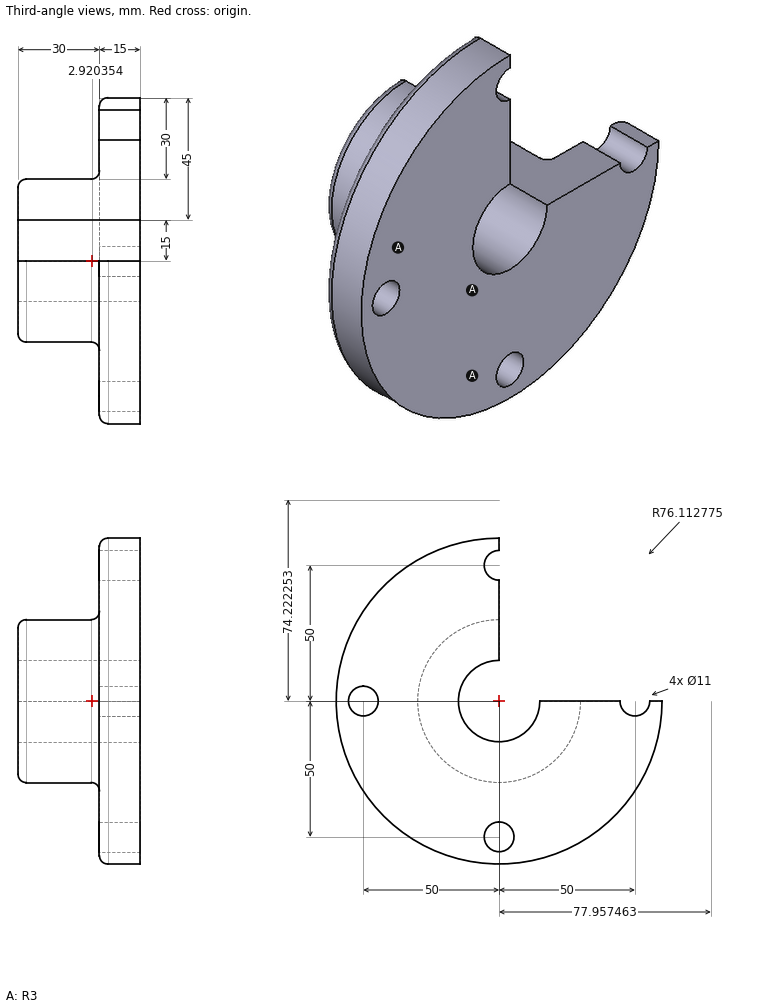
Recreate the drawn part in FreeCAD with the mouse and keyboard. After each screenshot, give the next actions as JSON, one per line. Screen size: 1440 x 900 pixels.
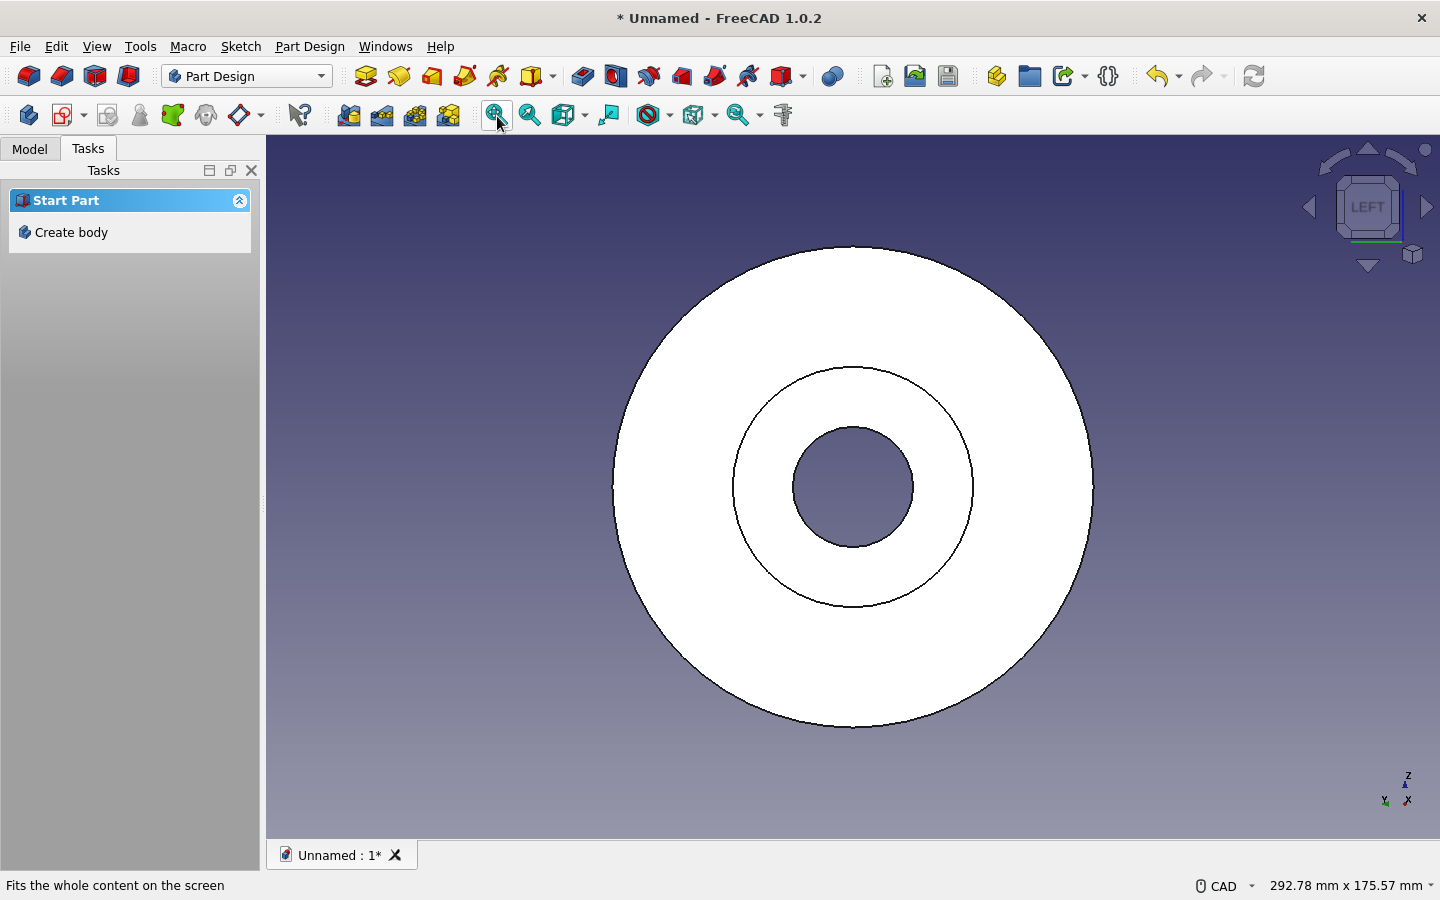
{"action": "left_click", "coordinate": [990, 623]}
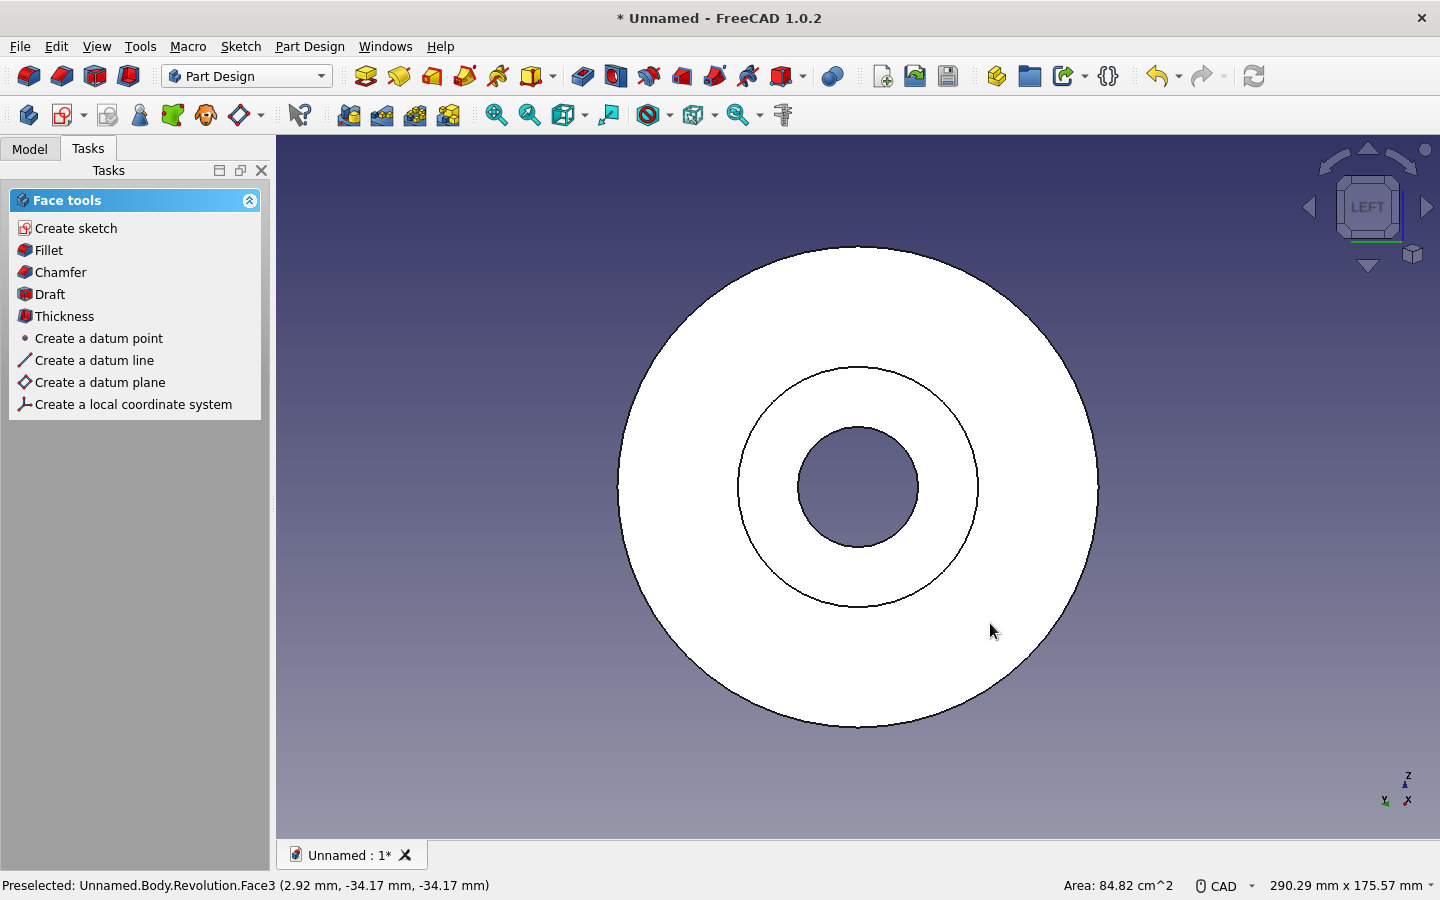
{"action": "left_click", "coordinate": [62, 116]}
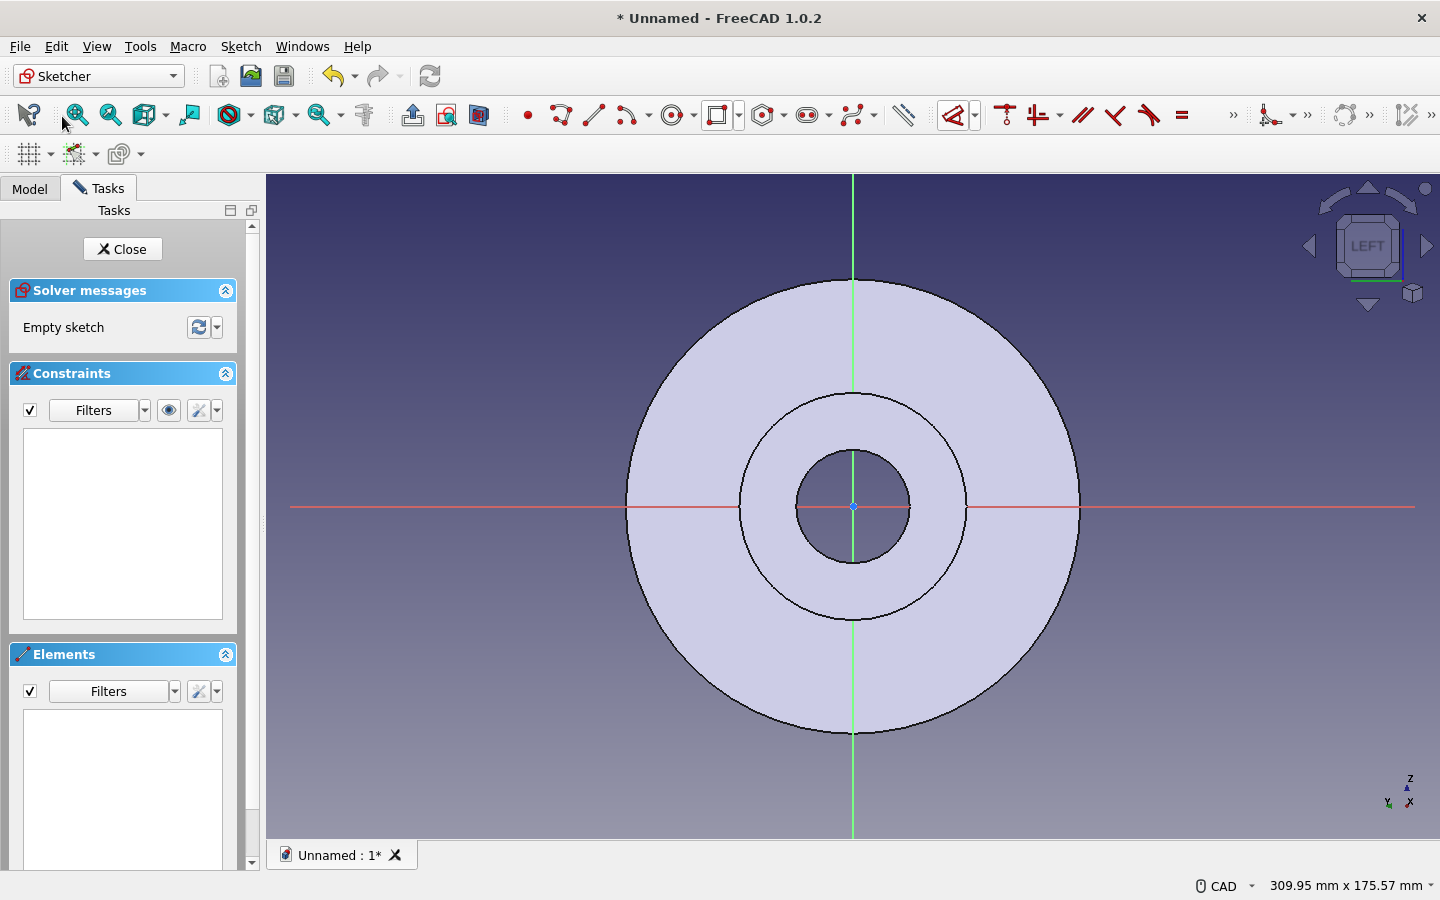
{"action": "left_click", "coordinate": [479, 116]}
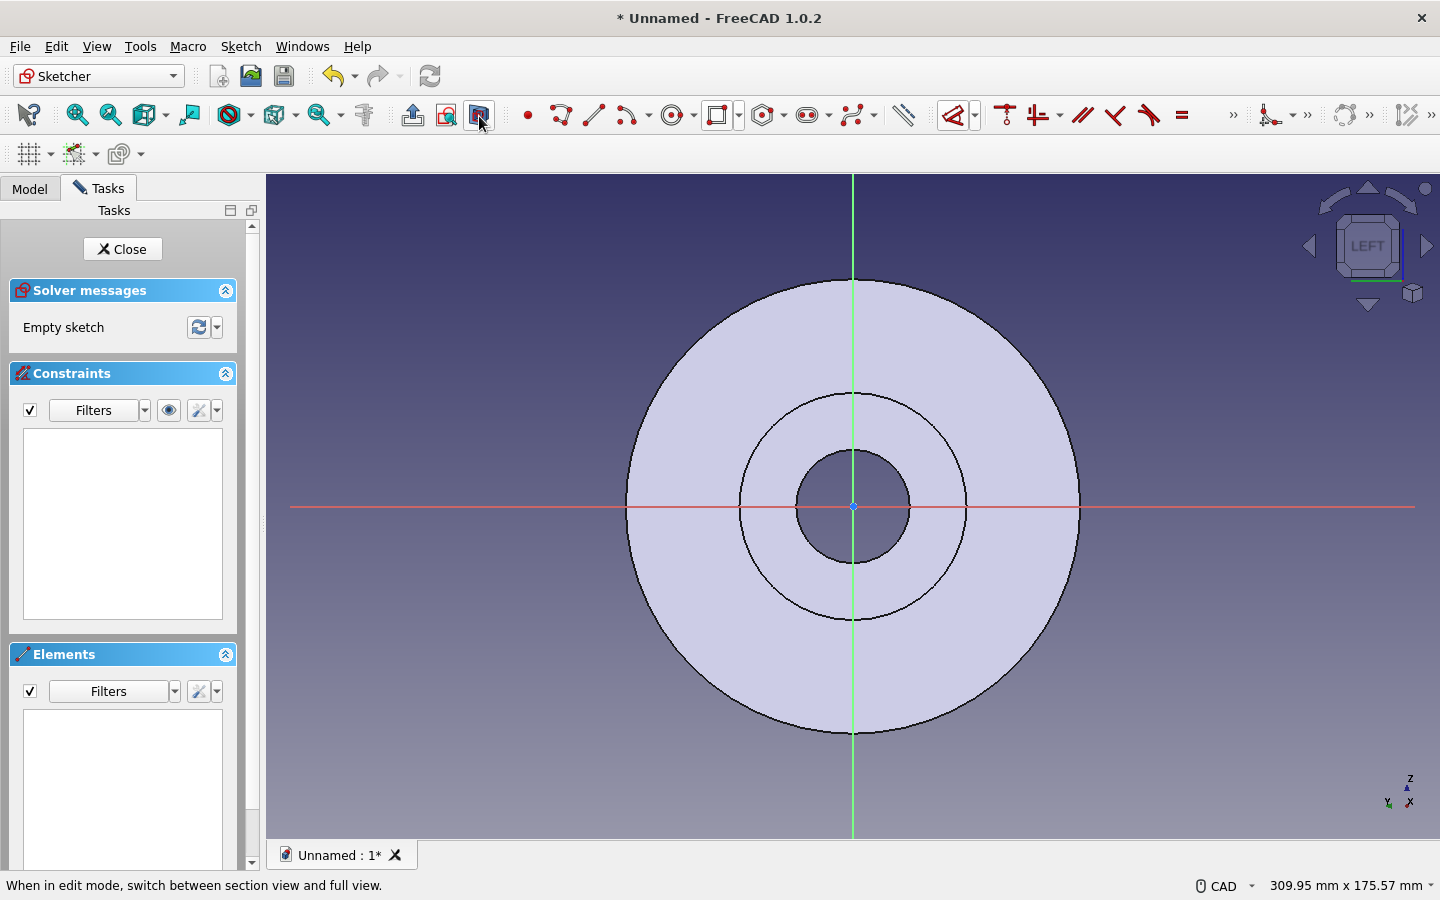
{"action": "left_click", "coordinate": [672, 116]}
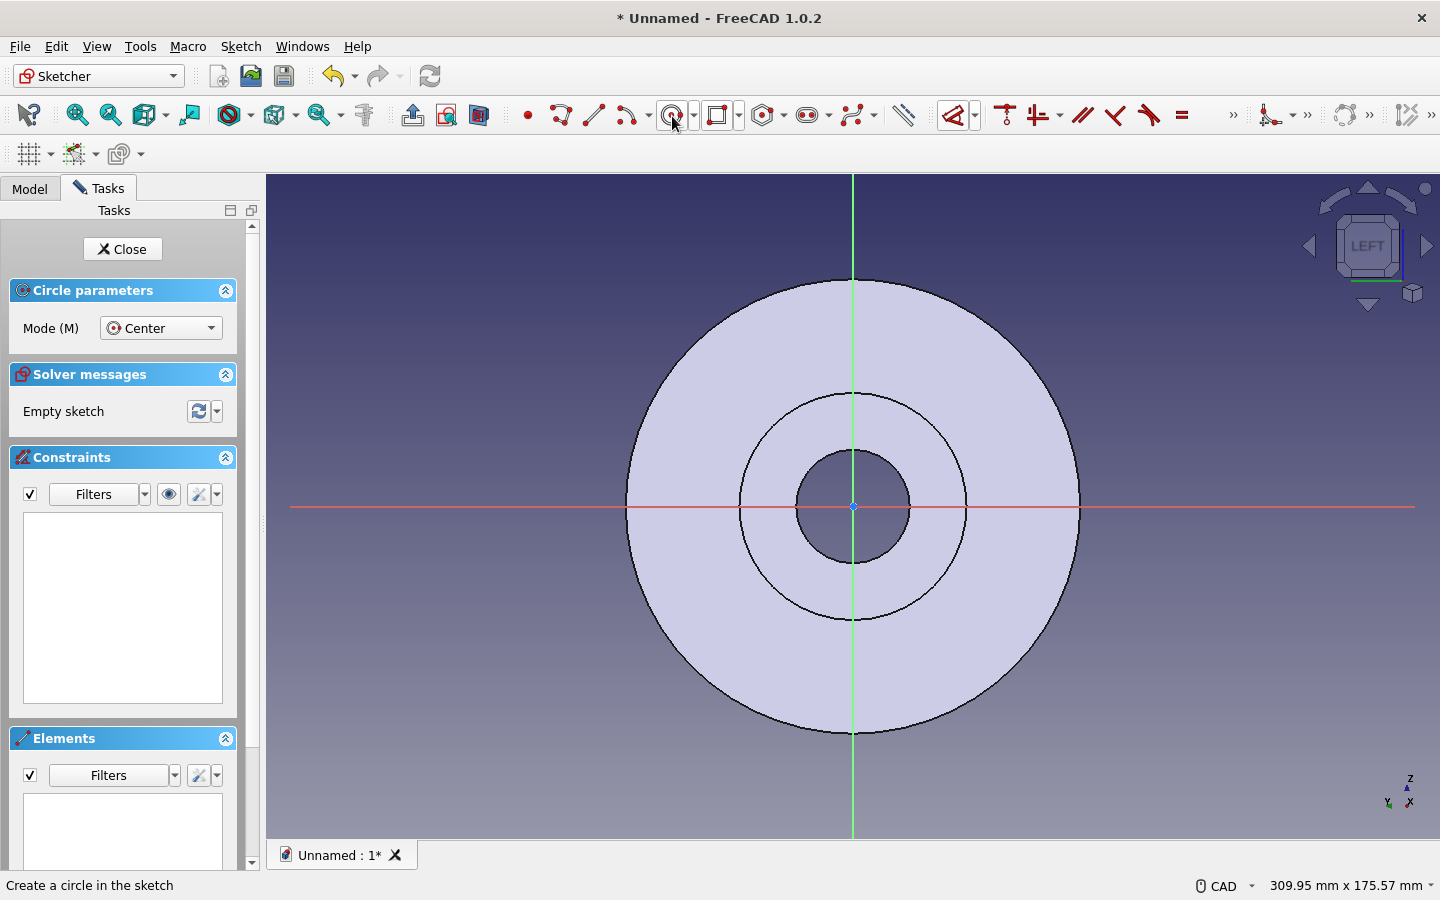
{"action": "left_click", "coordinate": [664, 506]}
{"action": "left_click", "coordinate": [678, 492]}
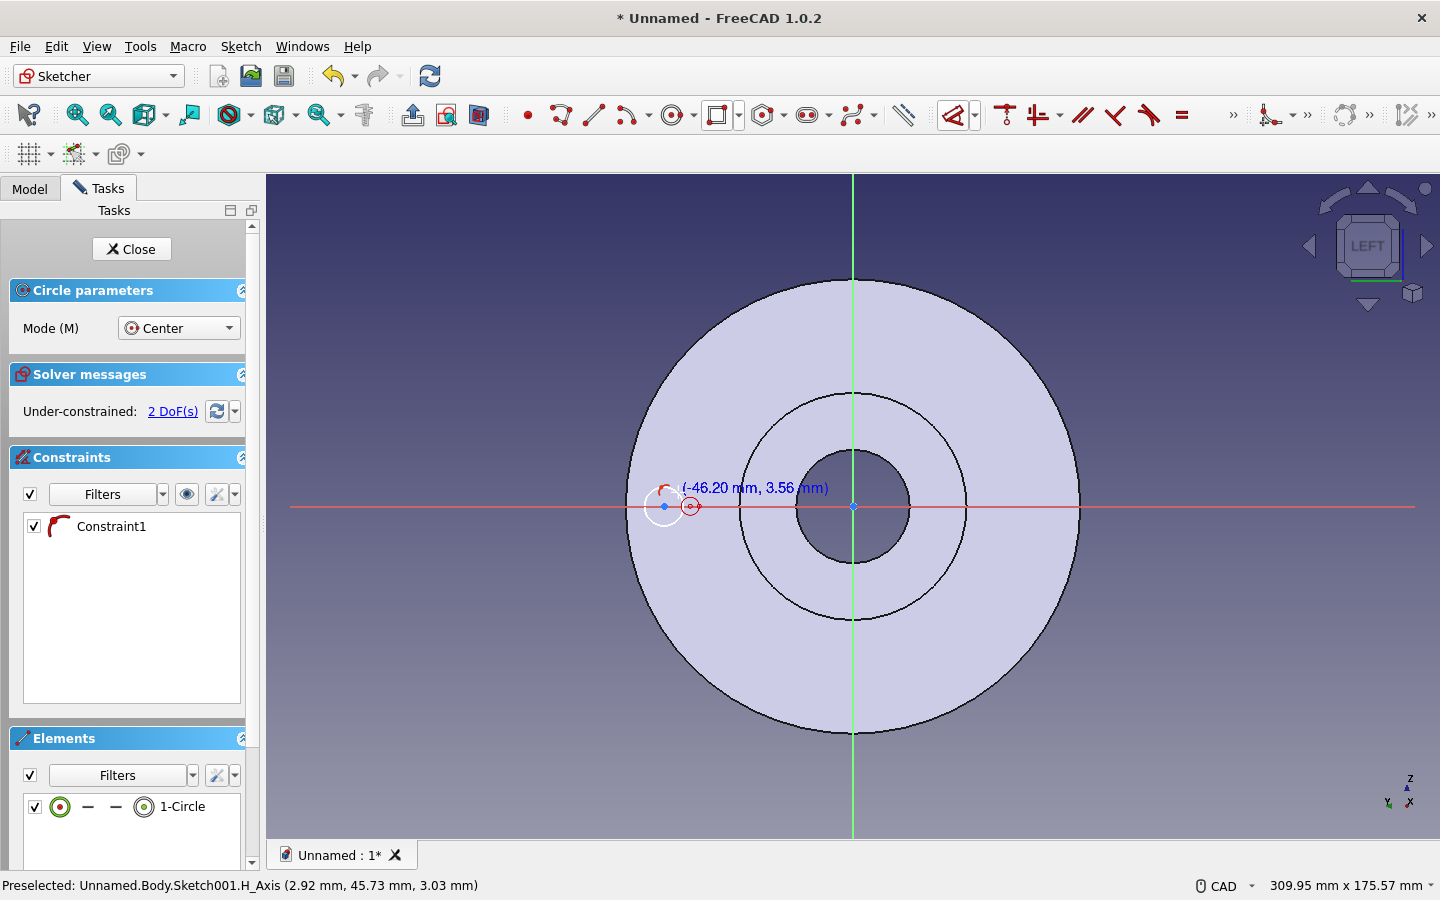
{"action": "left_click", "coordinate": [853, 317]}
{"action": "left_click", "coordinate": [868, 302]}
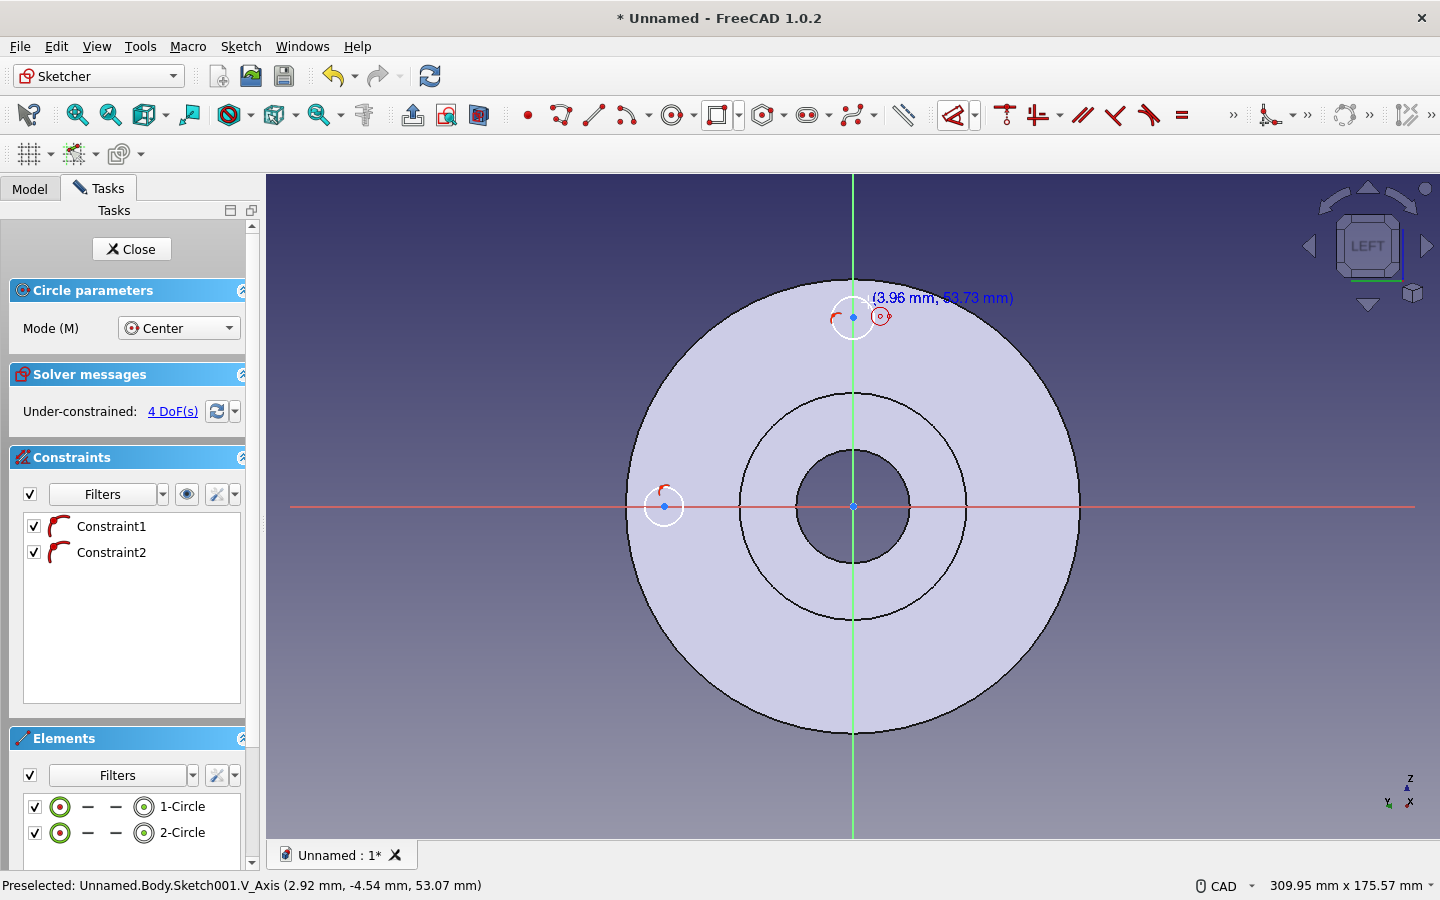
{"action": "left_click", "coordinate": [1042, 506]}
{"action": "left_click", "coordinate": [1057, 492]}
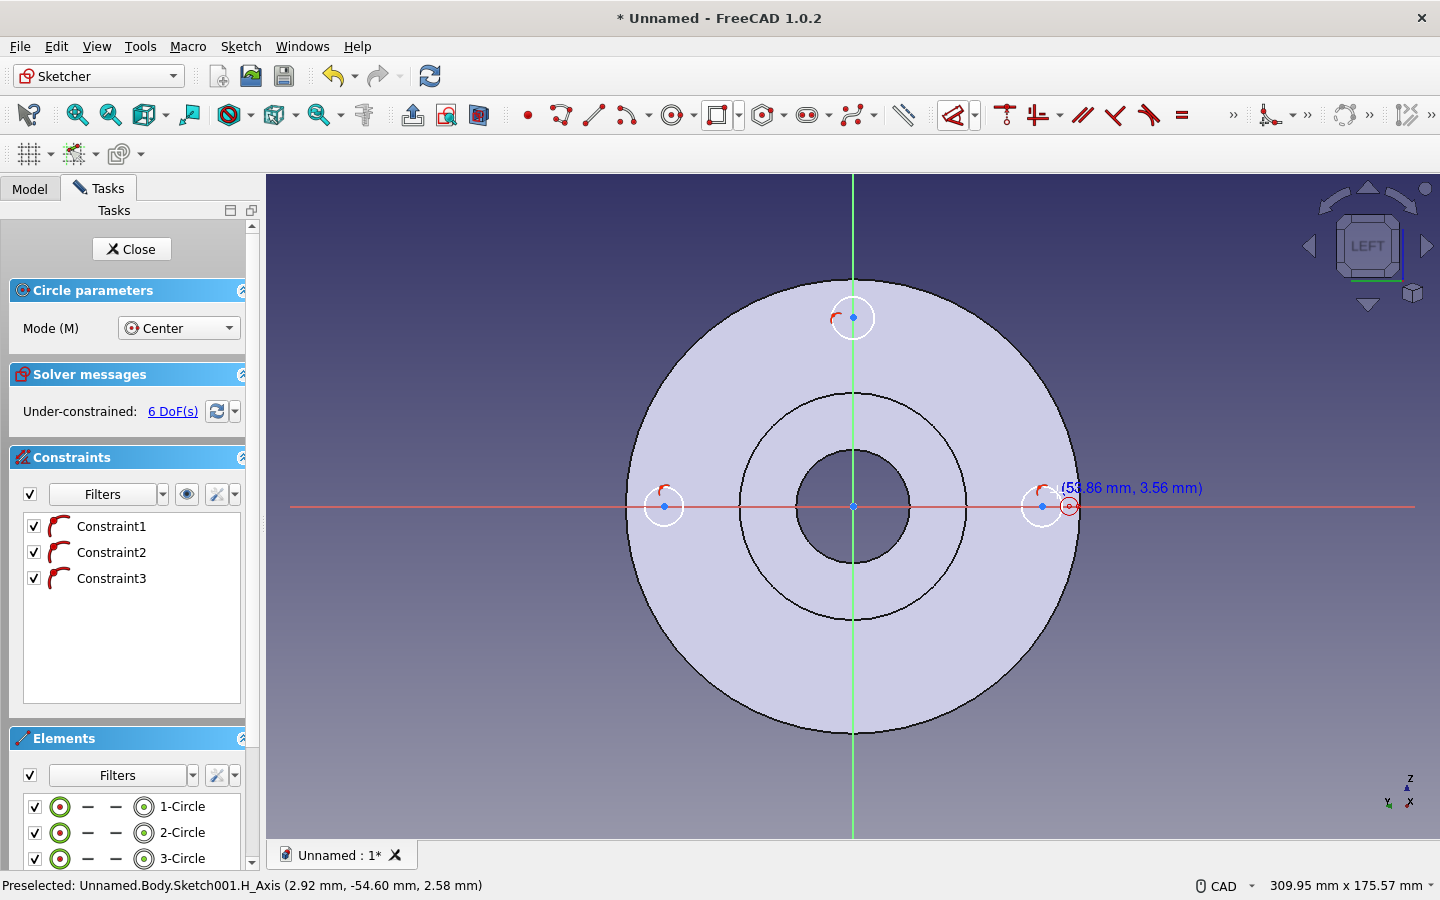
{"action": "left_click", "coordinate": [853, 696]}
{"action": "left_click", "coordinate": [868, 681]}
{"action": "key", "text": "Escape"}